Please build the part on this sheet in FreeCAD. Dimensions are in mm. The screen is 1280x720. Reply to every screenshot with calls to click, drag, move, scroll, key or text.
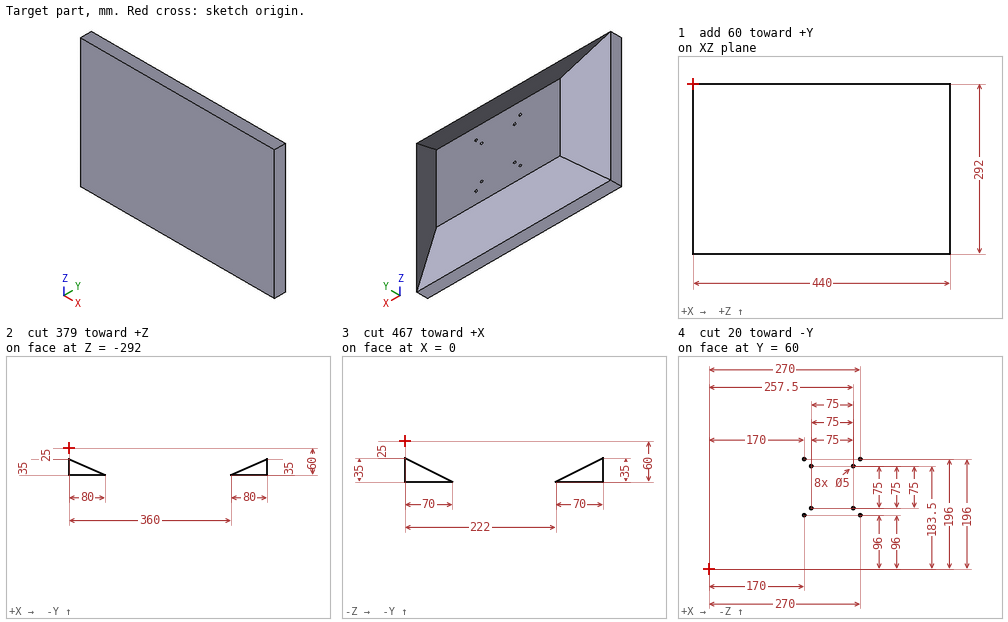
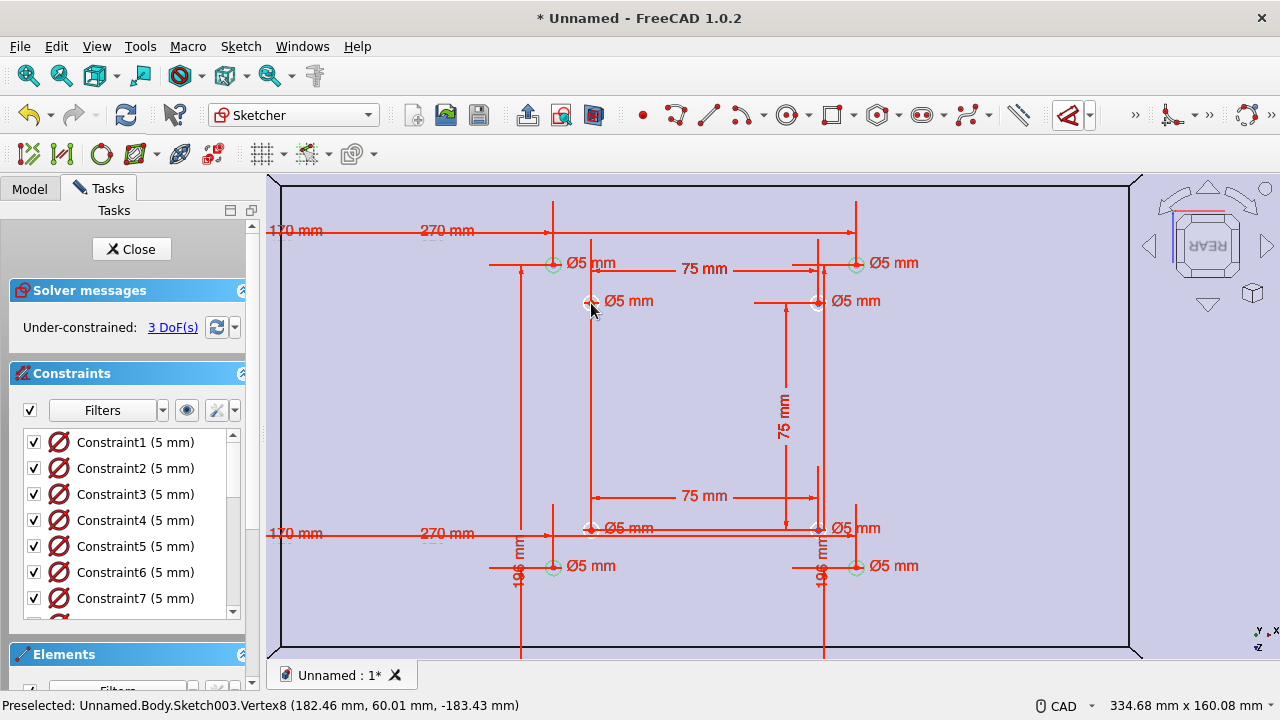
key(i)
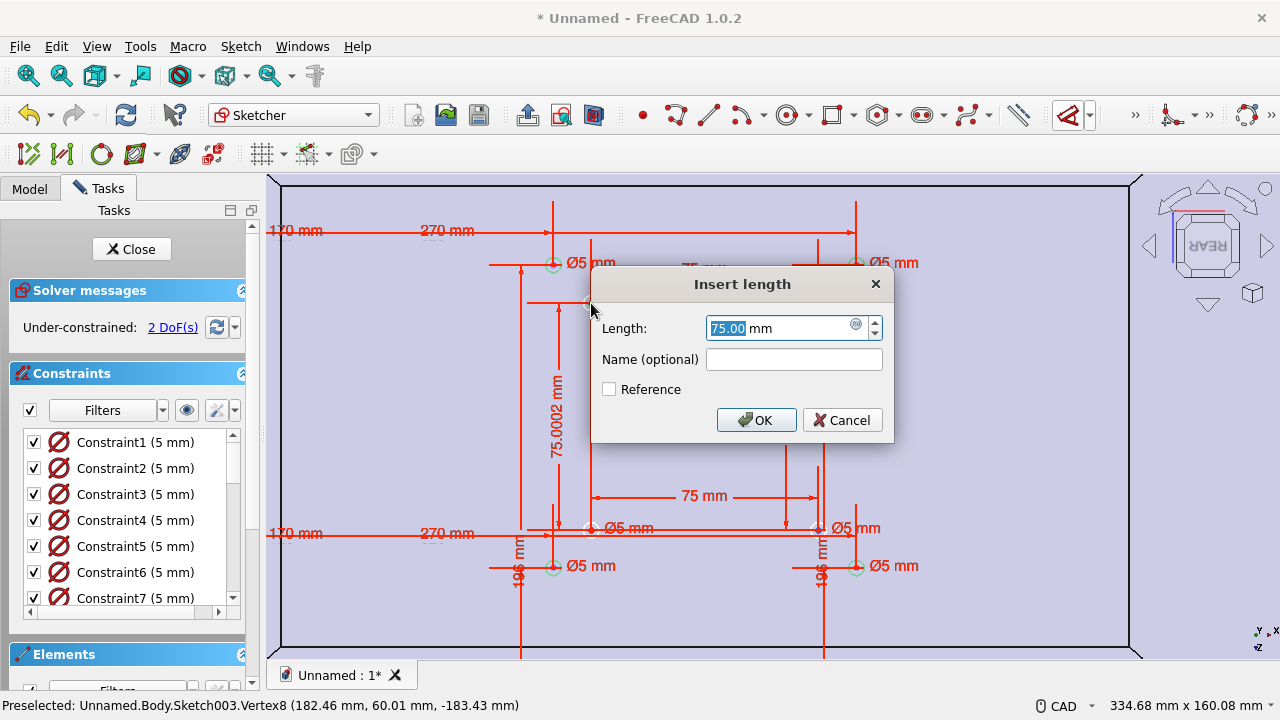
text(75)
key(Return)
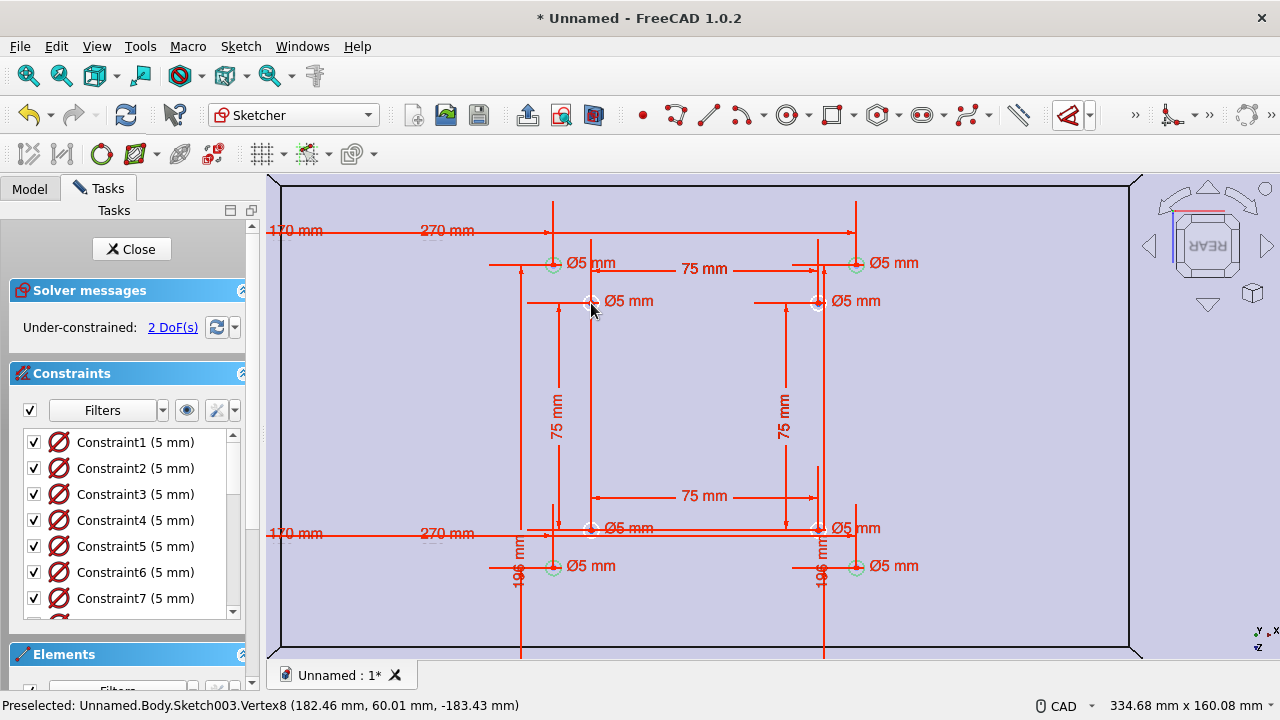
click(818, 303)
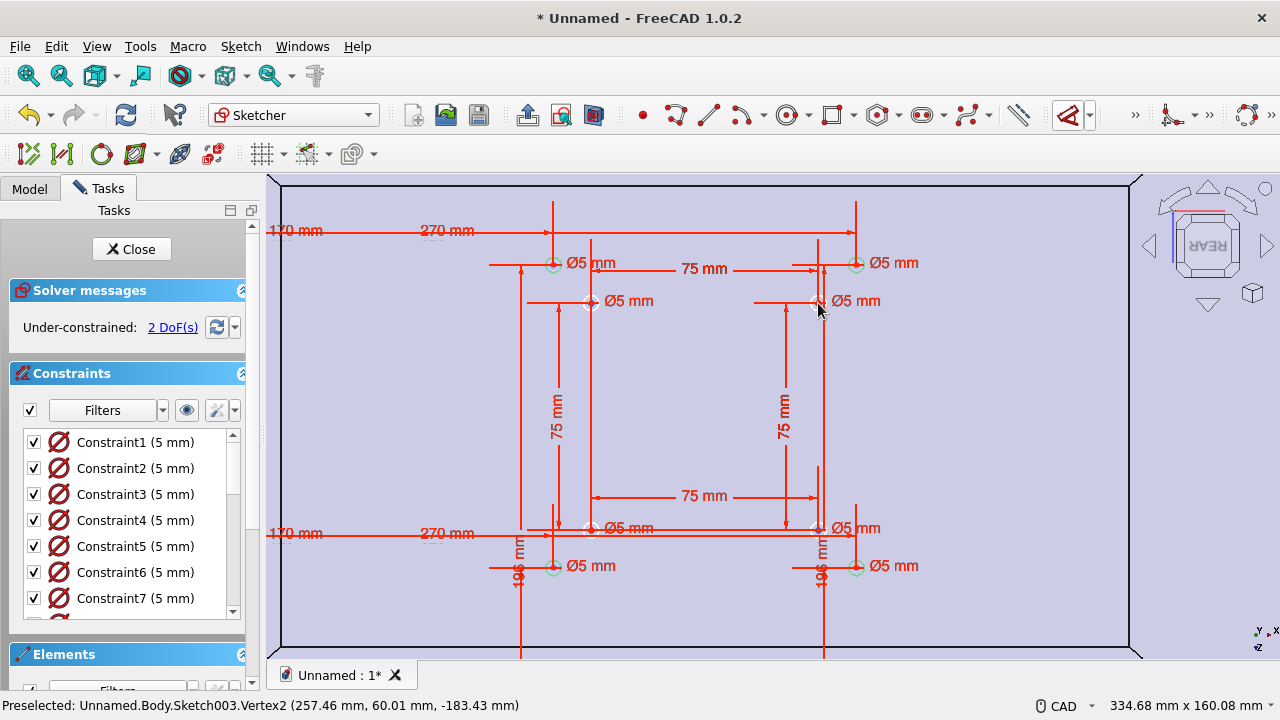
click(1090, 116)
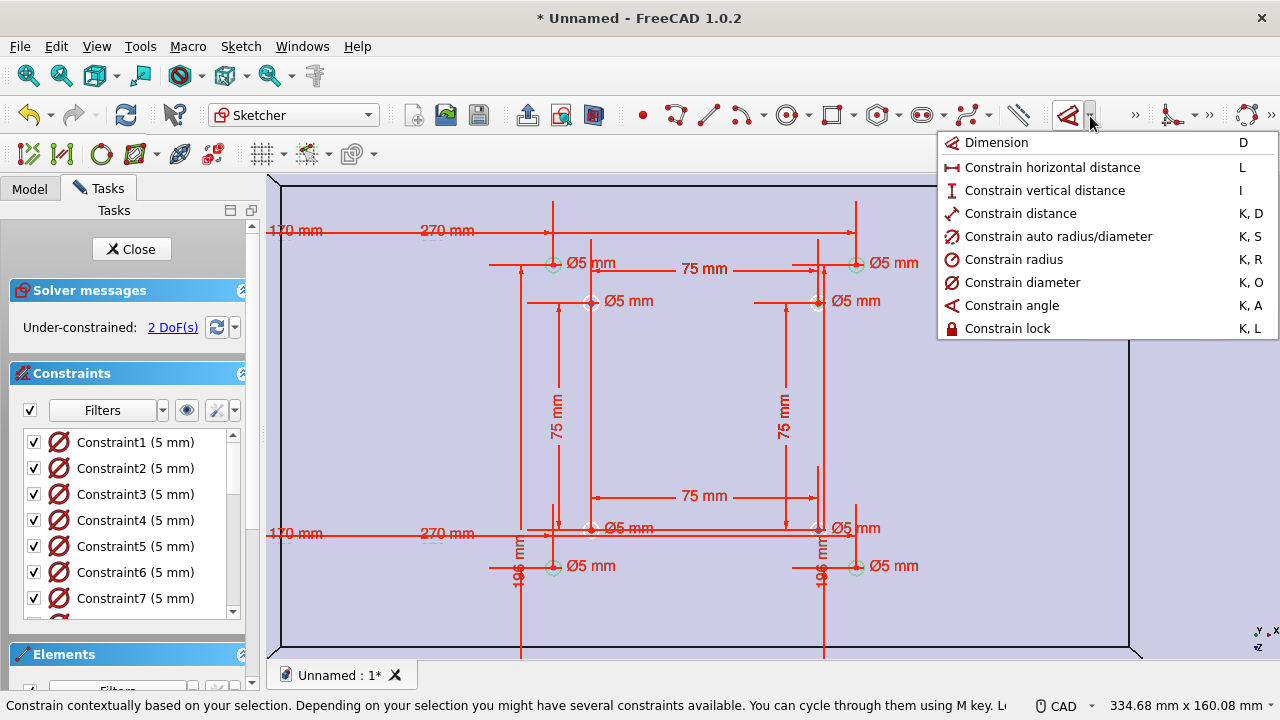
click(1108, 168)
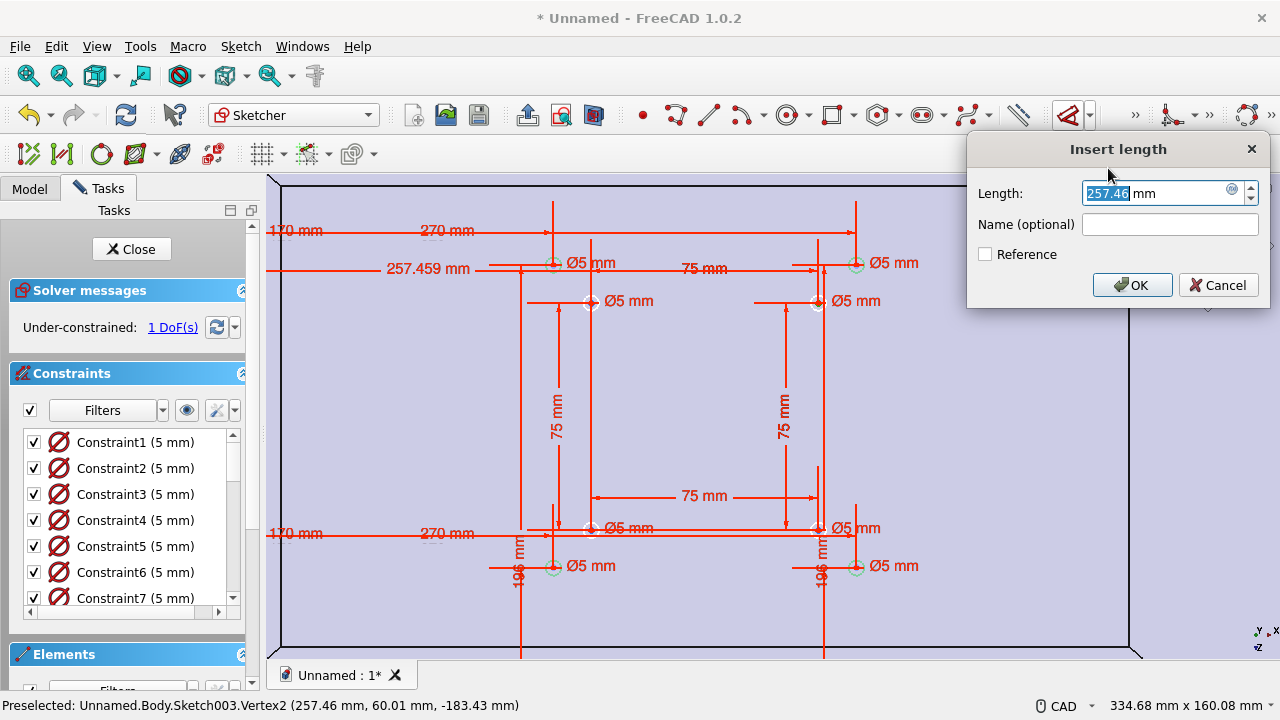
text(257.5)
key(Return)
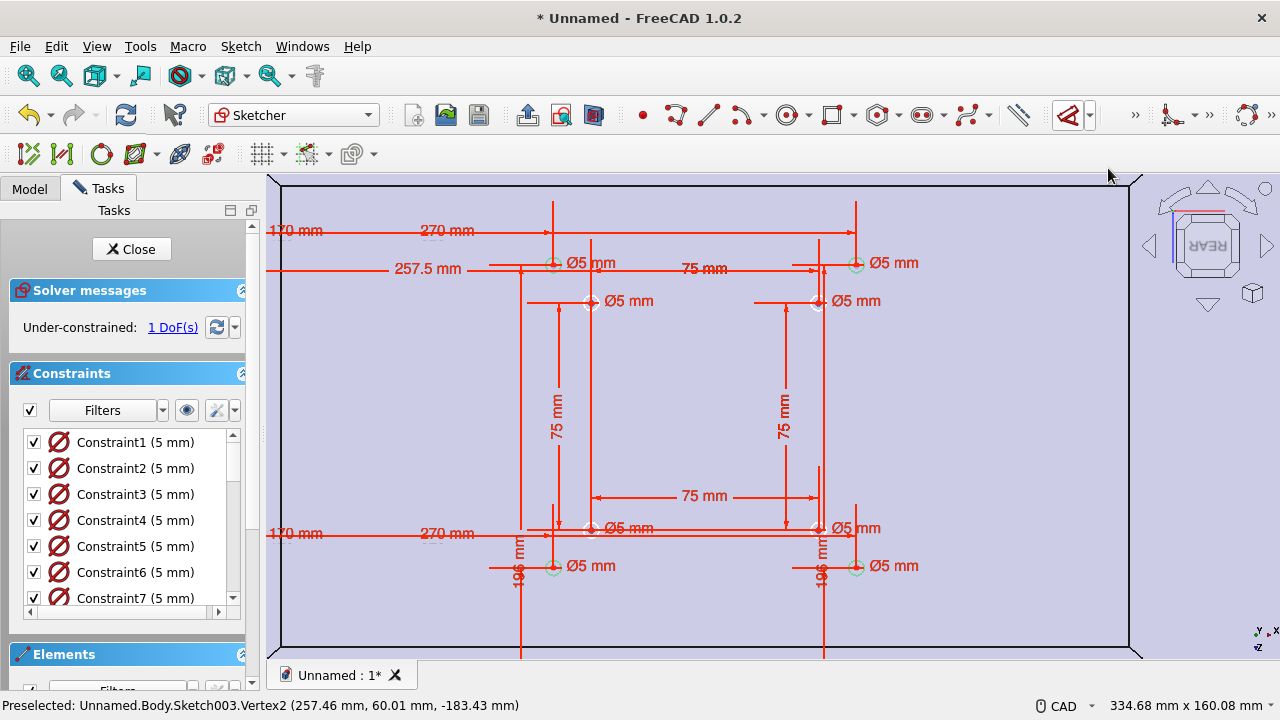
click(819, 303)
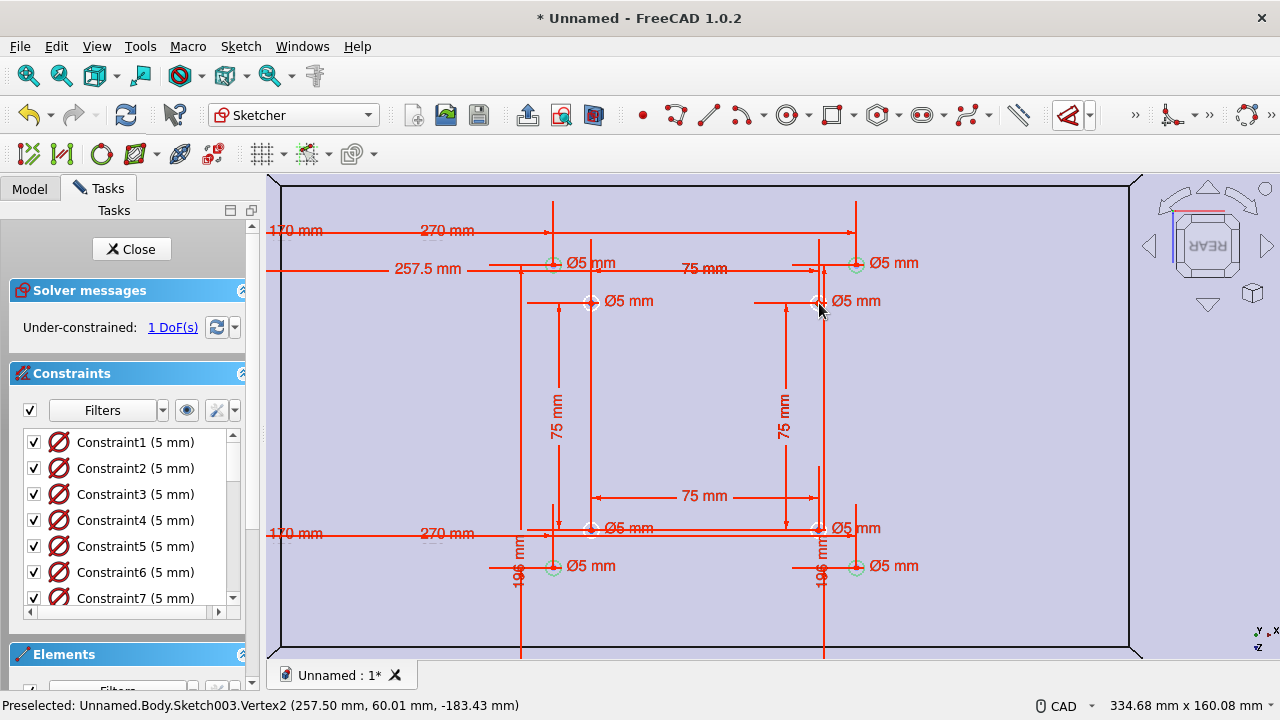
key(i)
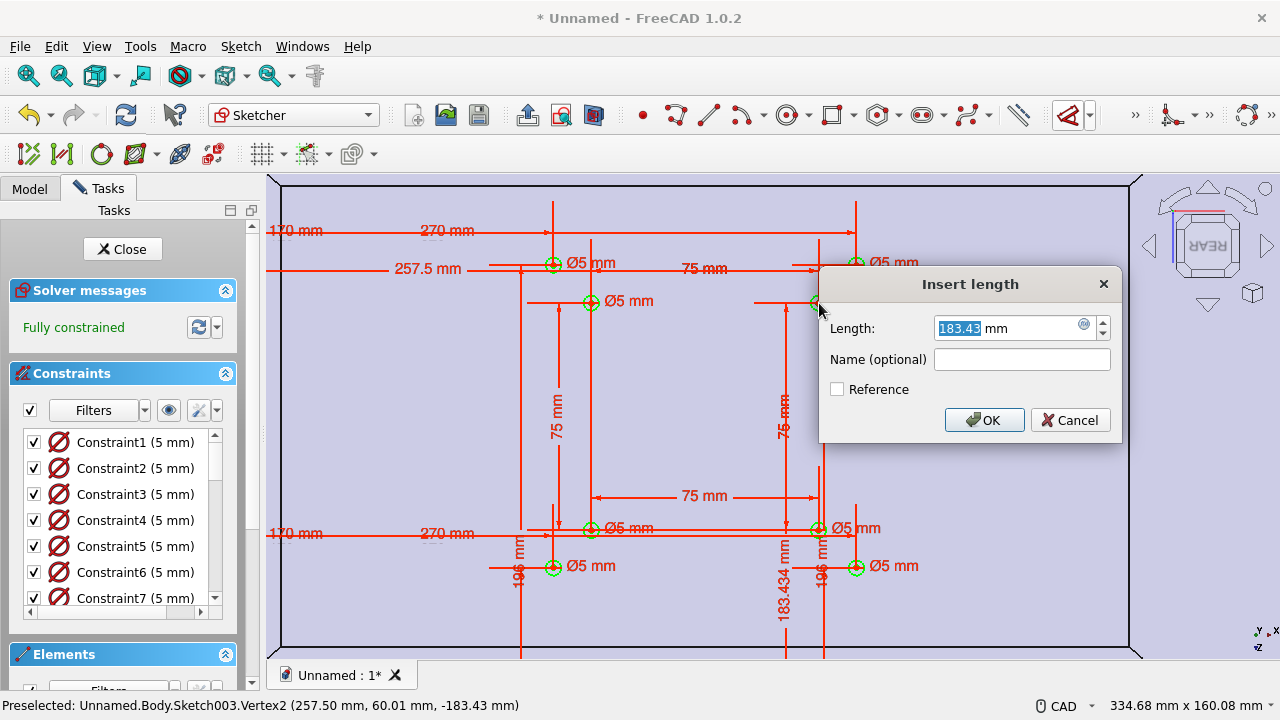
text(183.5)
key(Return)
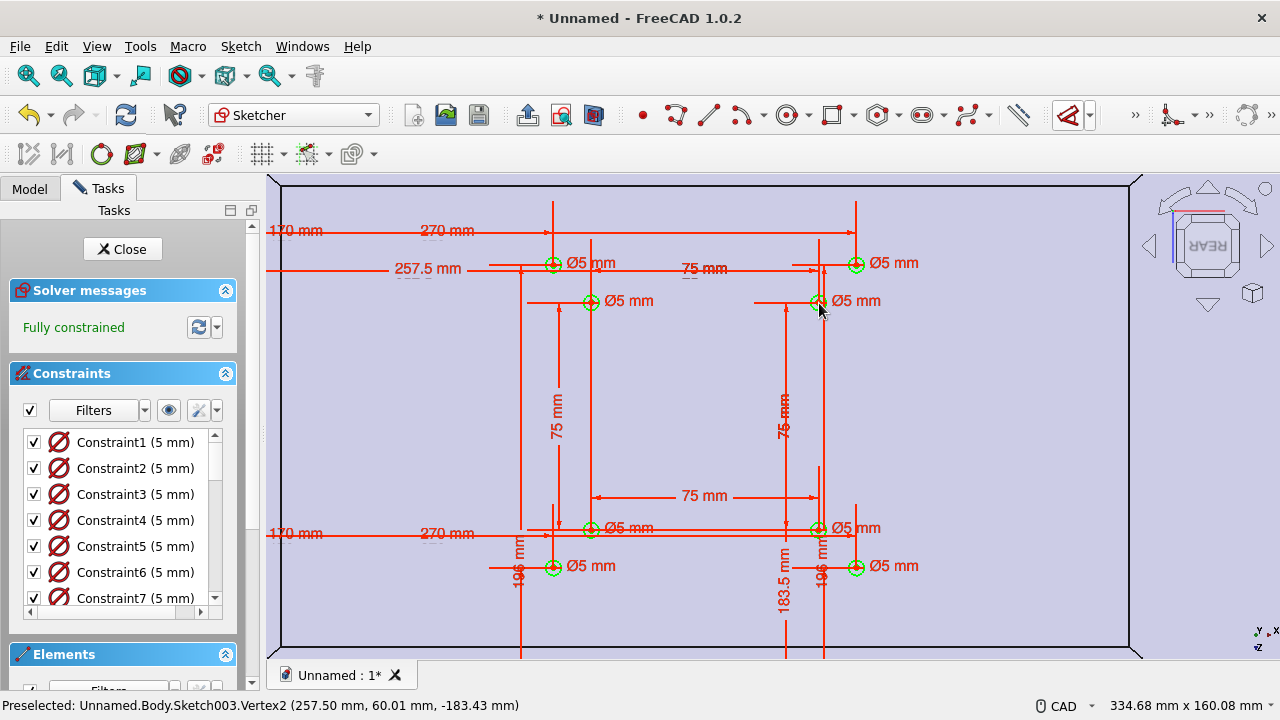
click(123, 249)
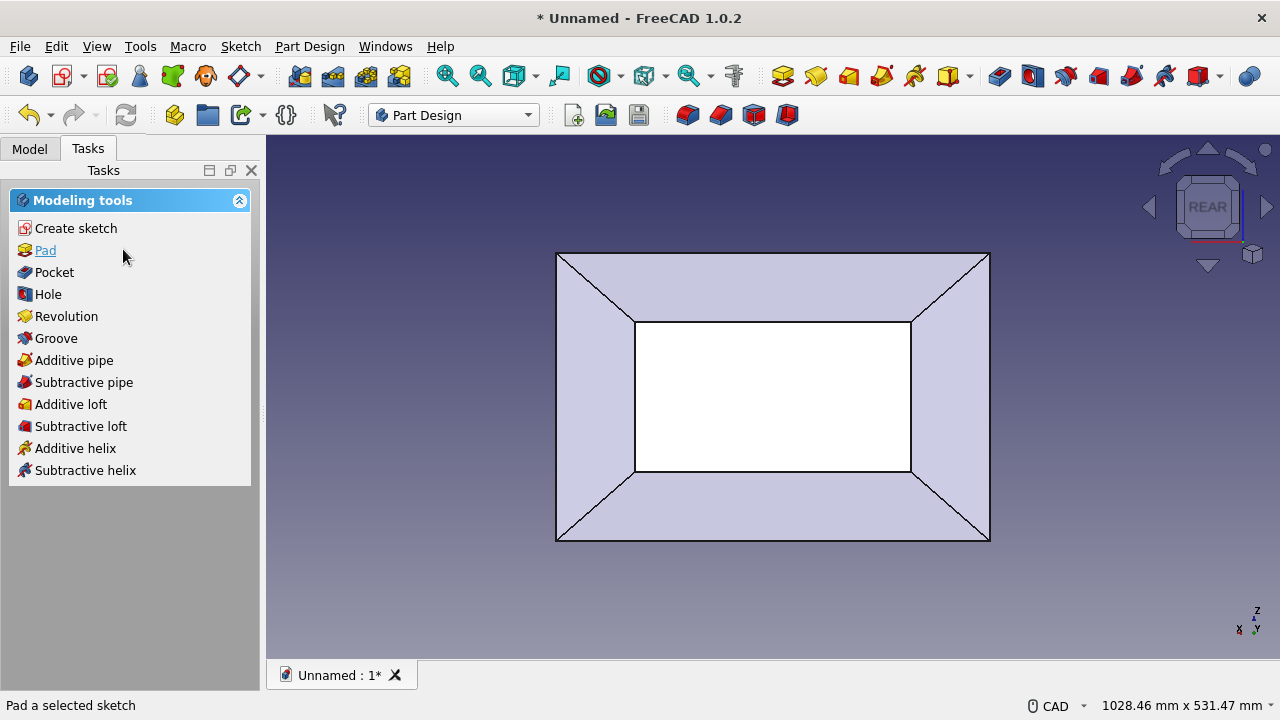
click(1000, 76)